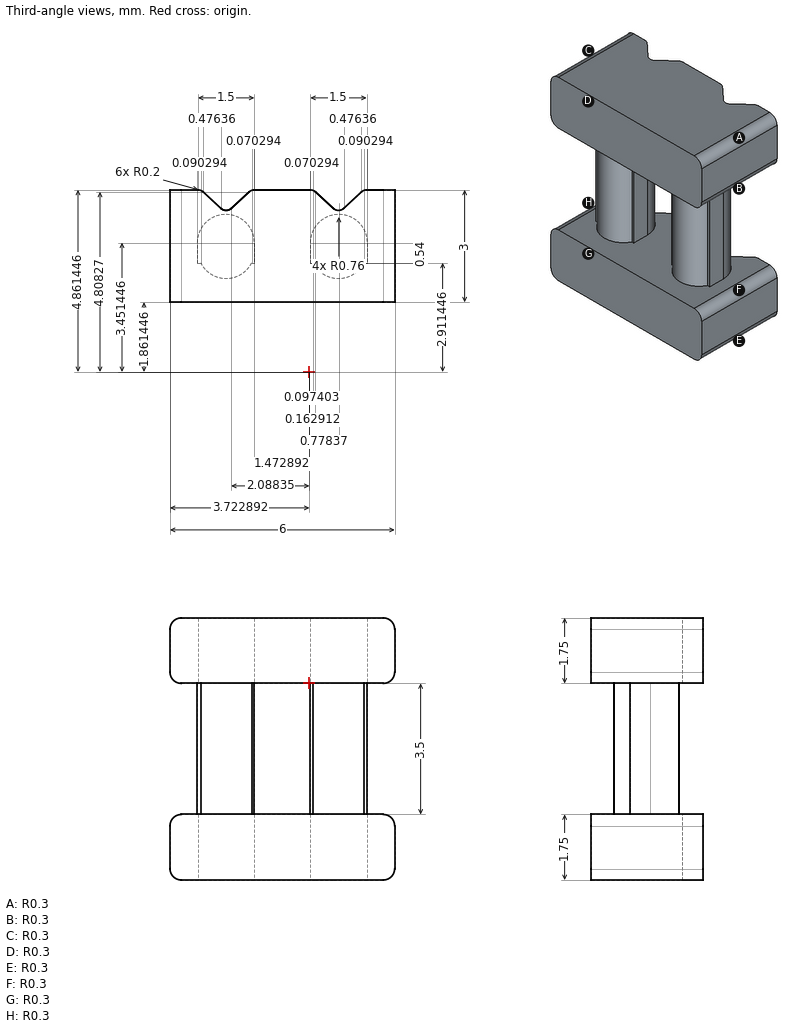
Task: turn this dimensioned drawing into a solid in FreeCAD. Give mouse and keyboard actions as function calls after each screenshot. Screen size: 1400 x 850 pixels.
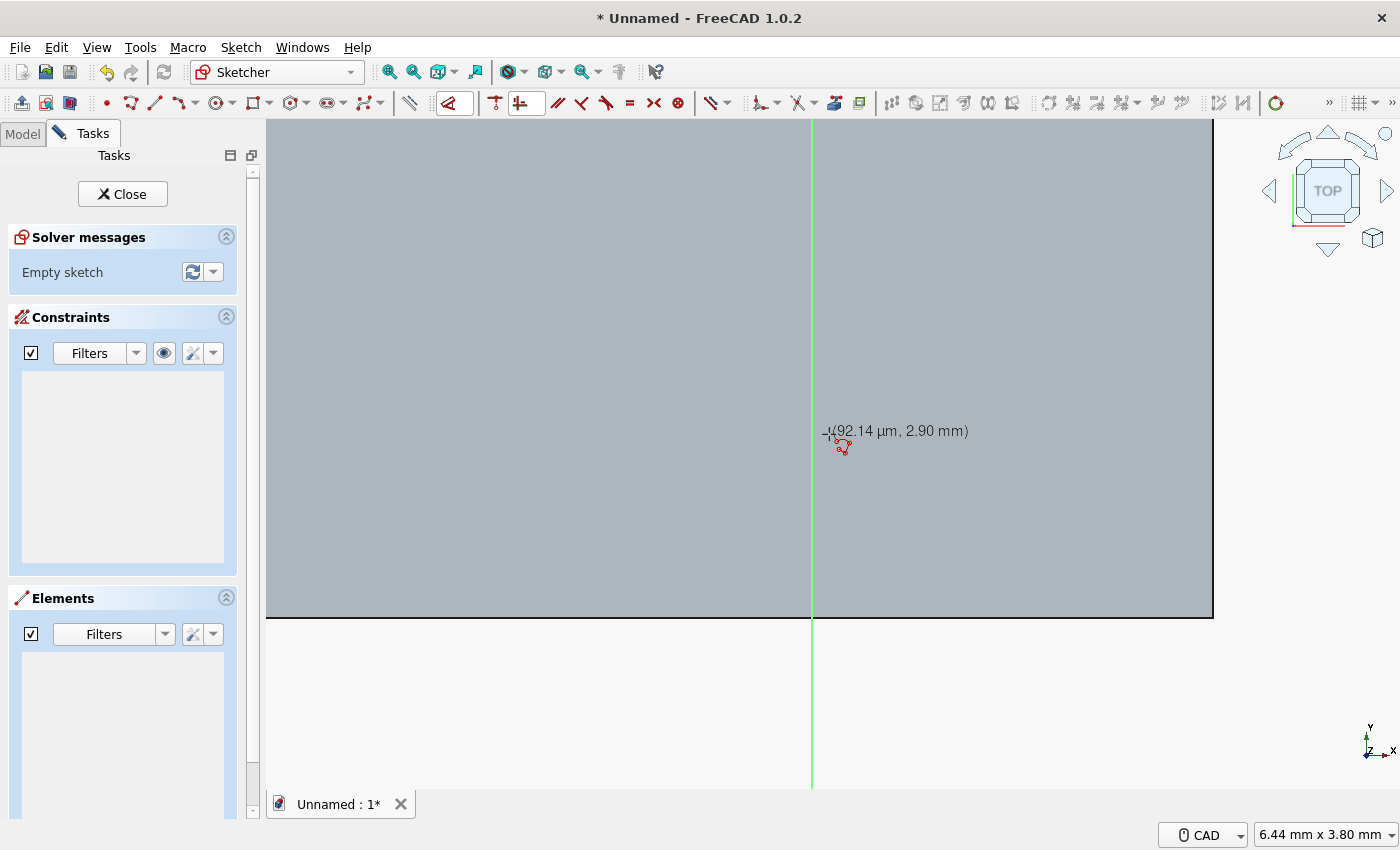
click(829, 433)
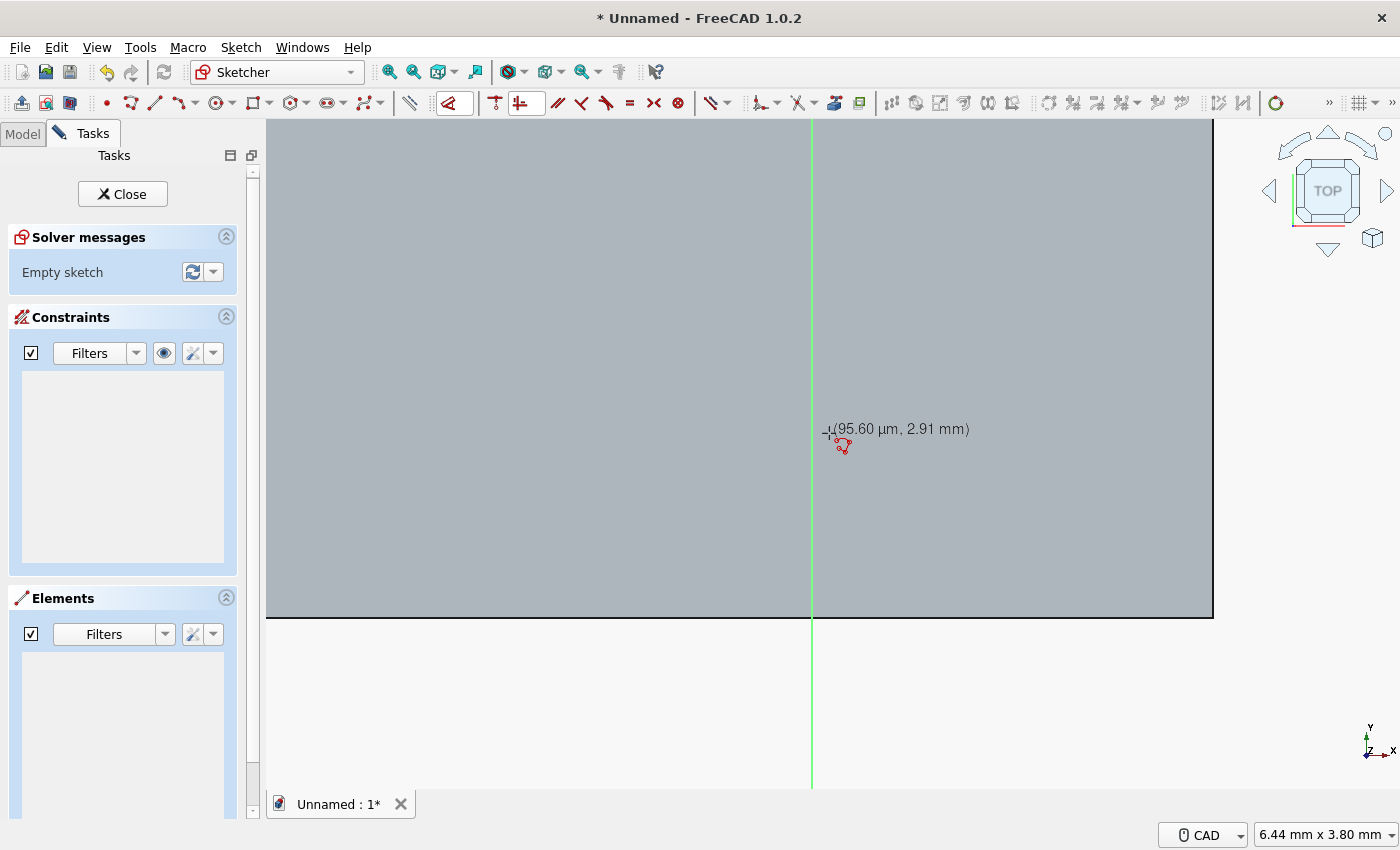
scroll(817, 433, up, 7)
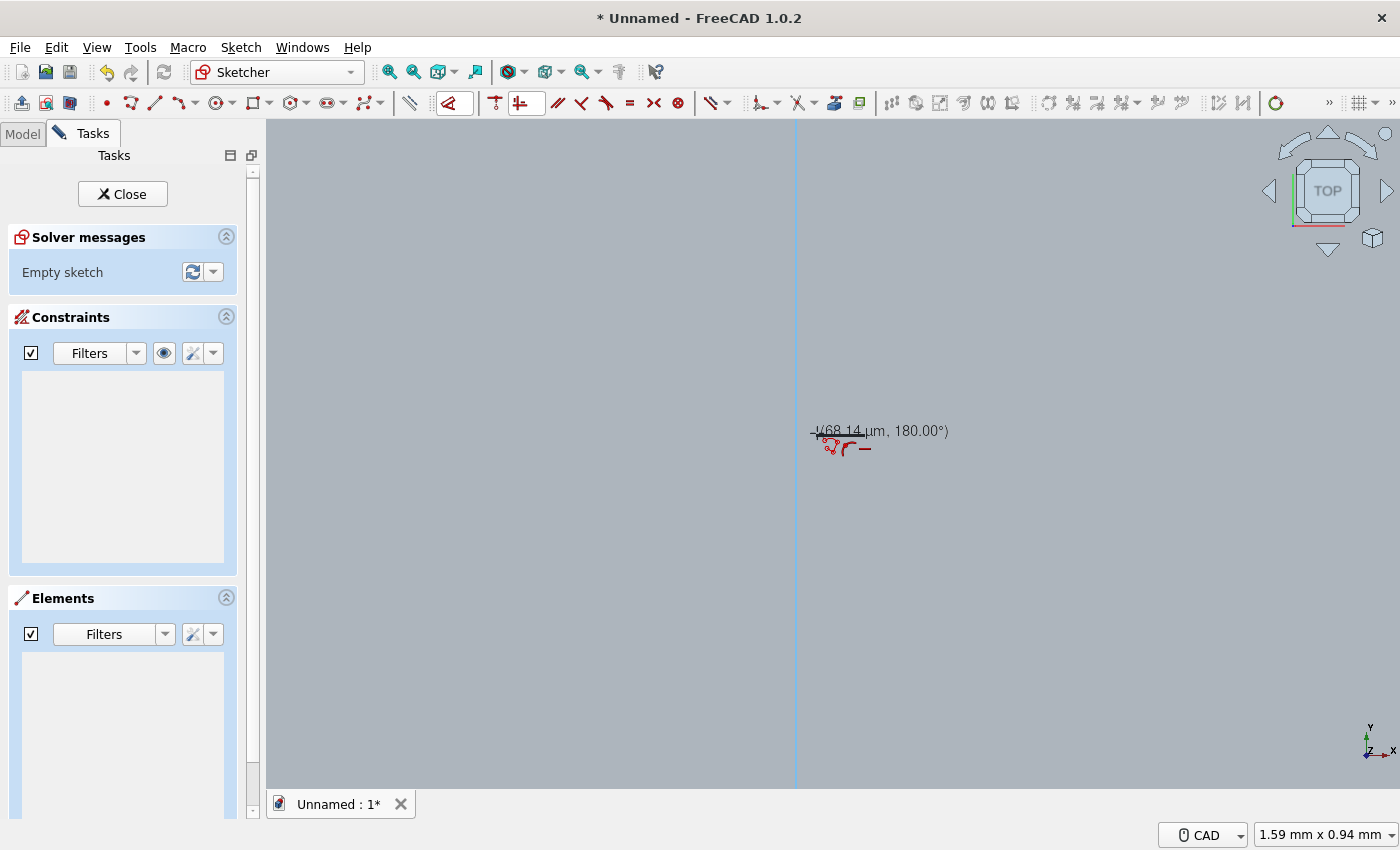
click(815, 432)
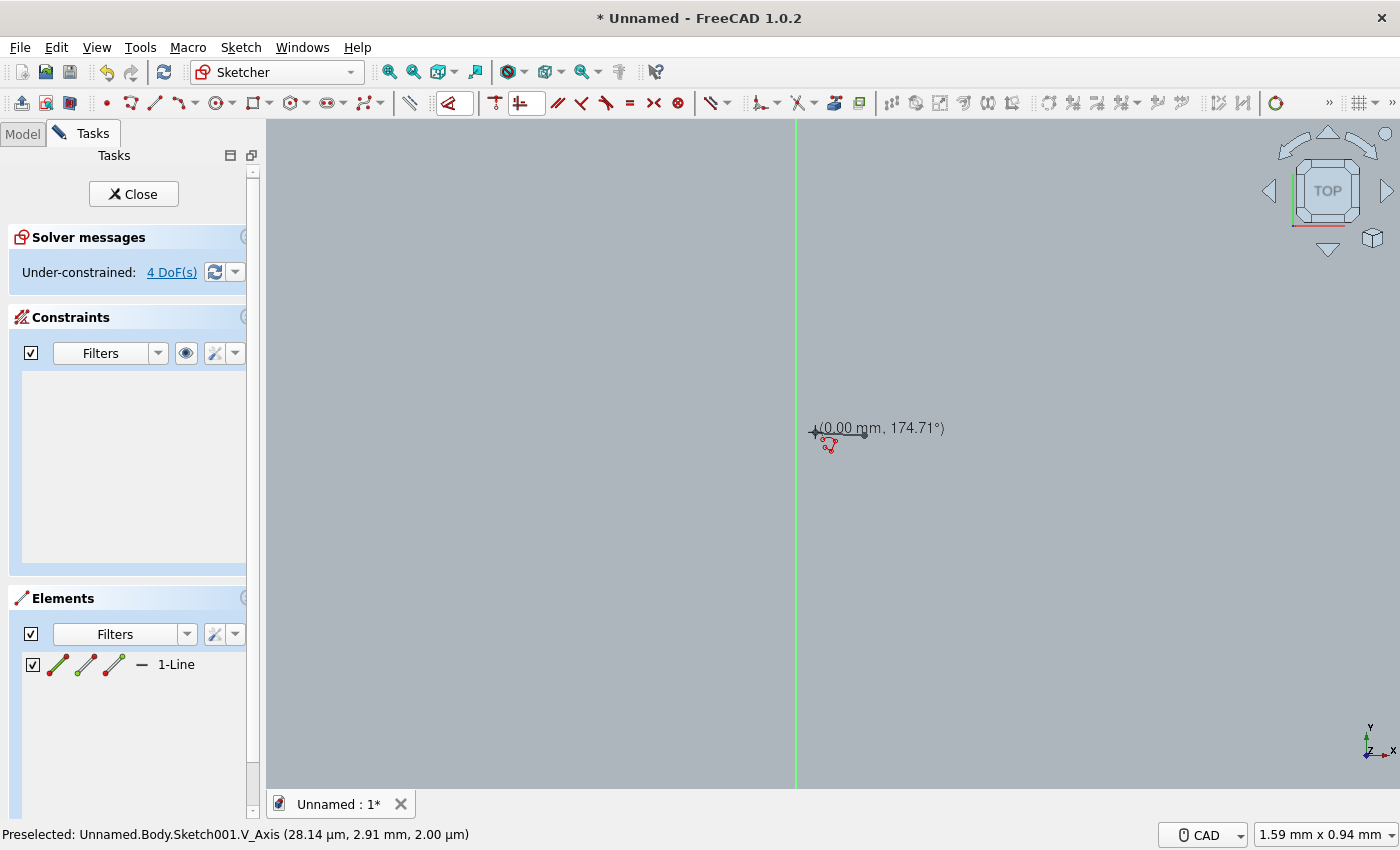
scroll(840, 367, down, 10)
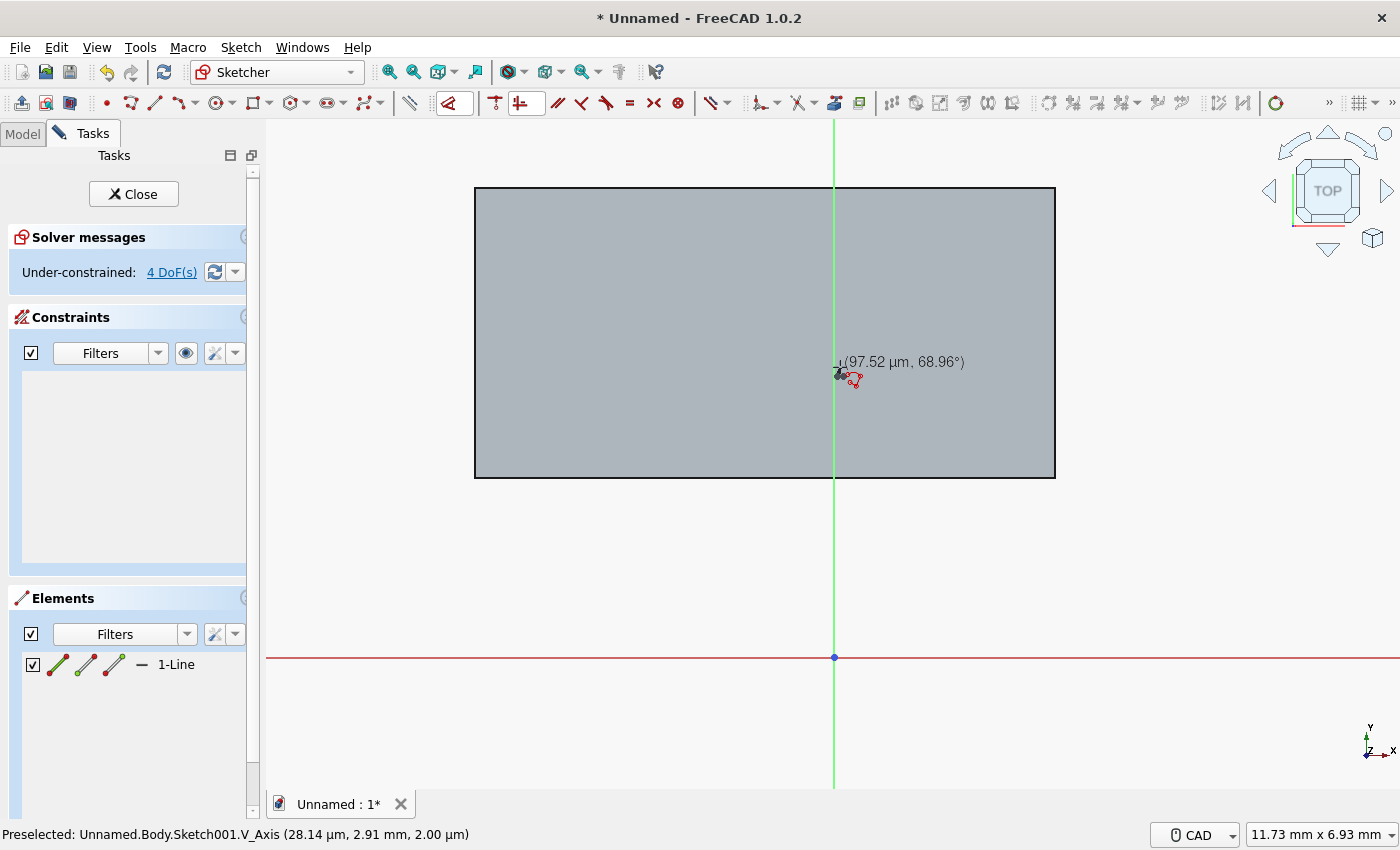
scroll(837, 324, up, 10)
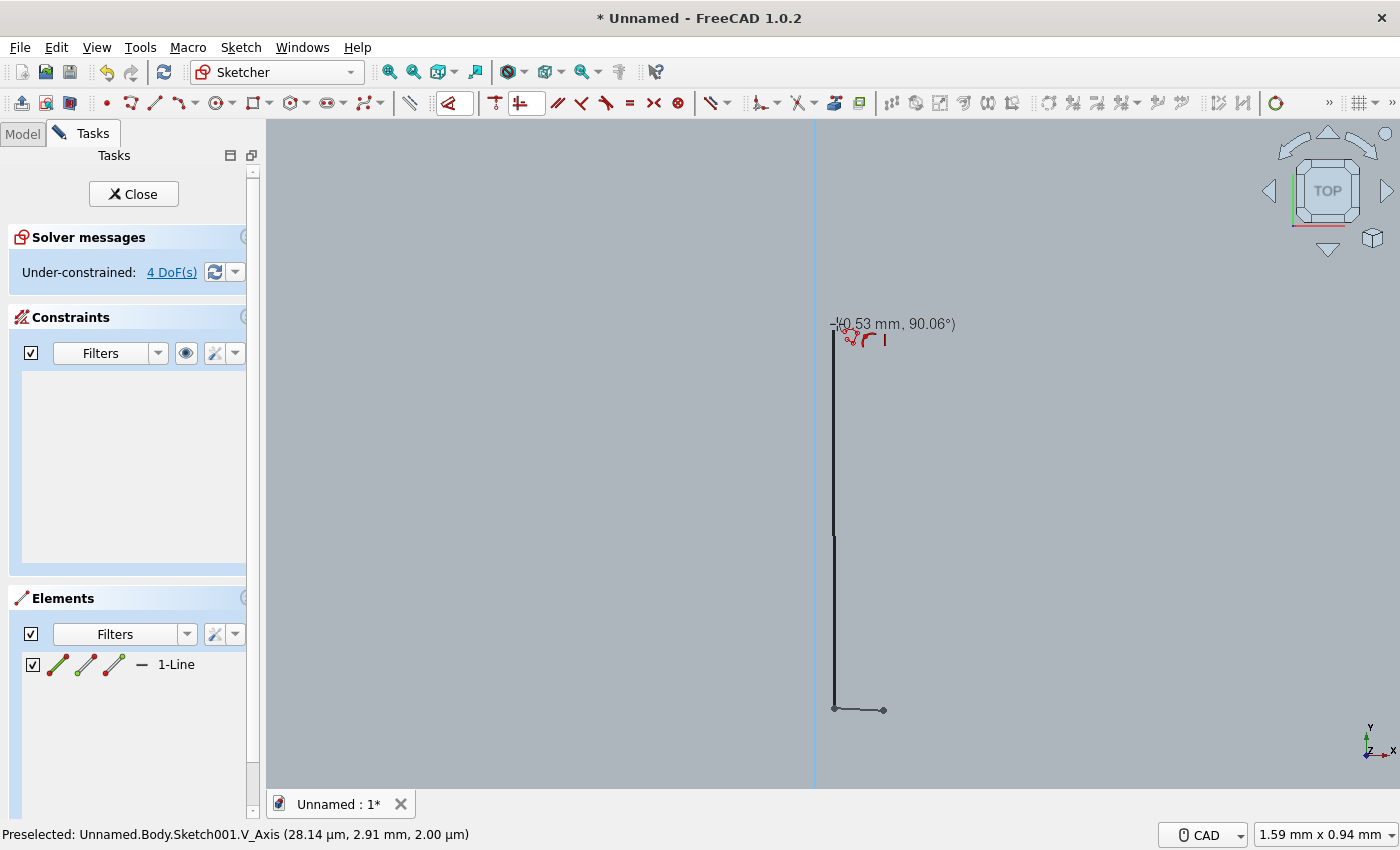
click(834, 322)
right_click(834, 322)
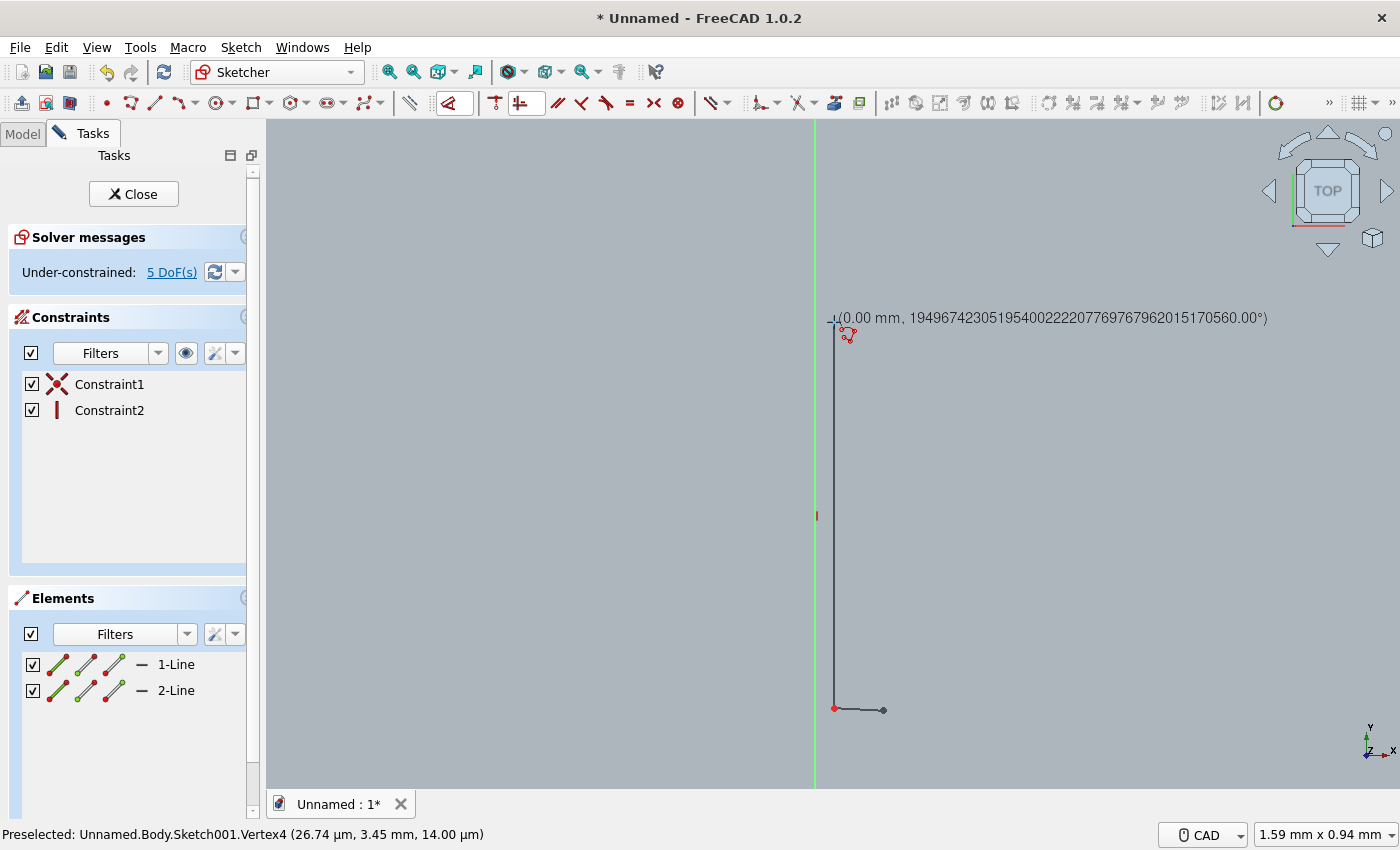
scroll(837, 324, down, 10)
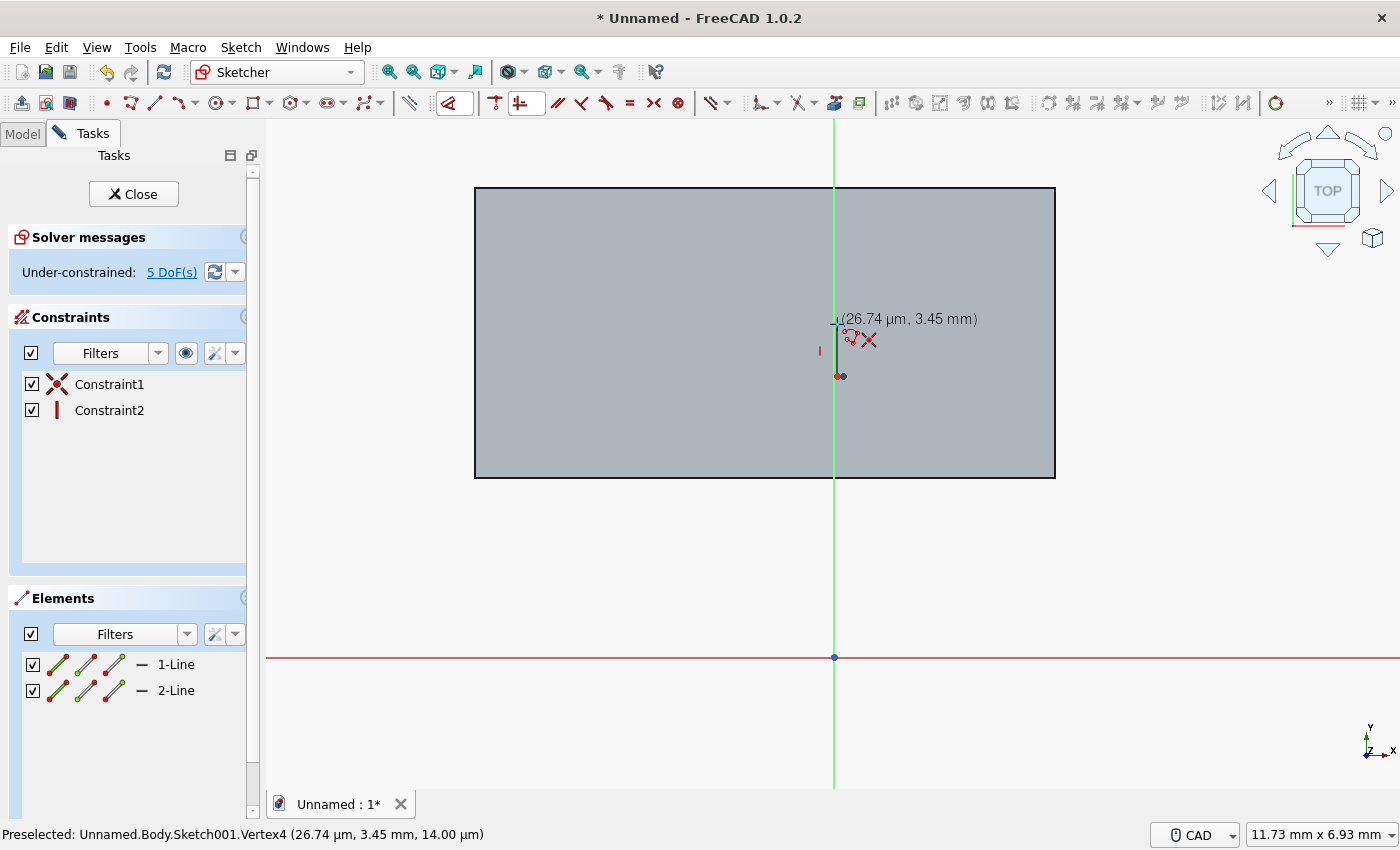
click(984, 324)
click(984, 376)